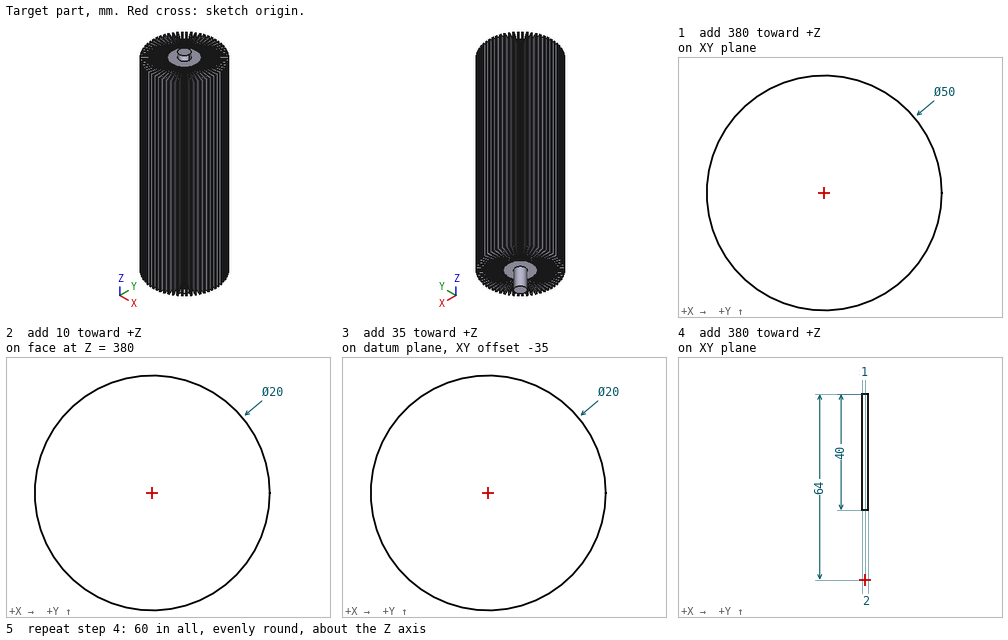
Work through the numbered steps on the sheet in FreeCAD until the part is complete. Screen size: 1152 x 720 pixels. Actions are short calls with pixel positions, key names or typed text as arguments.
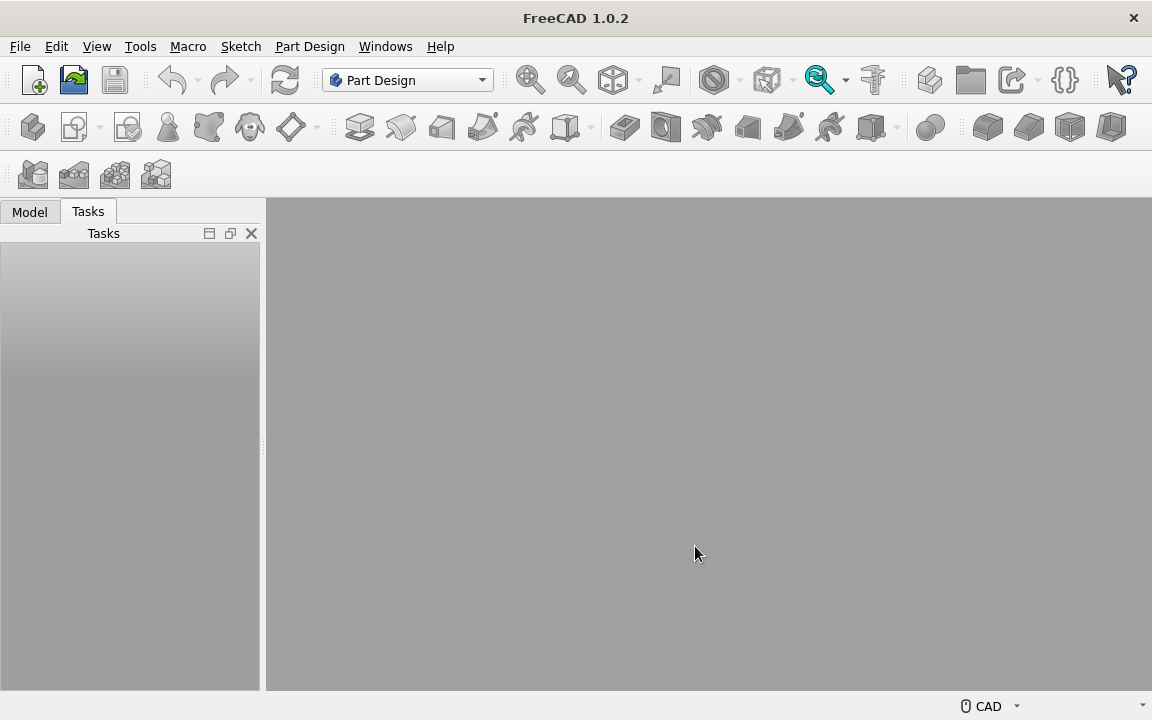
click(33, 80)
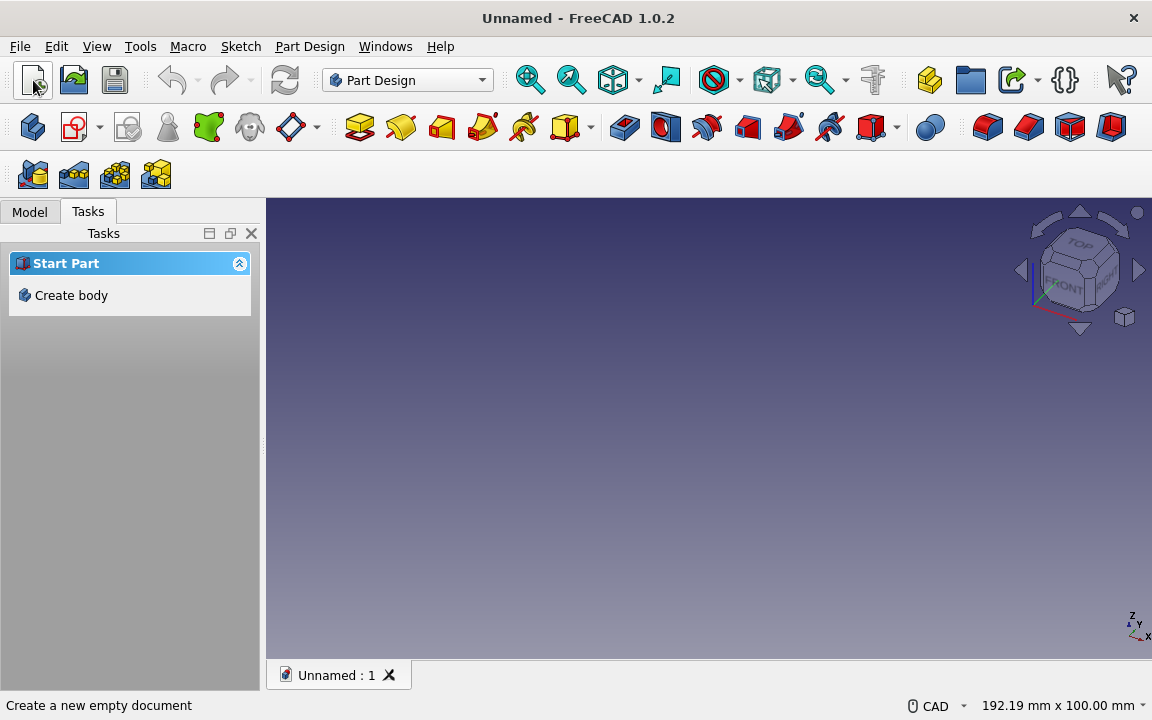
click(74, 128)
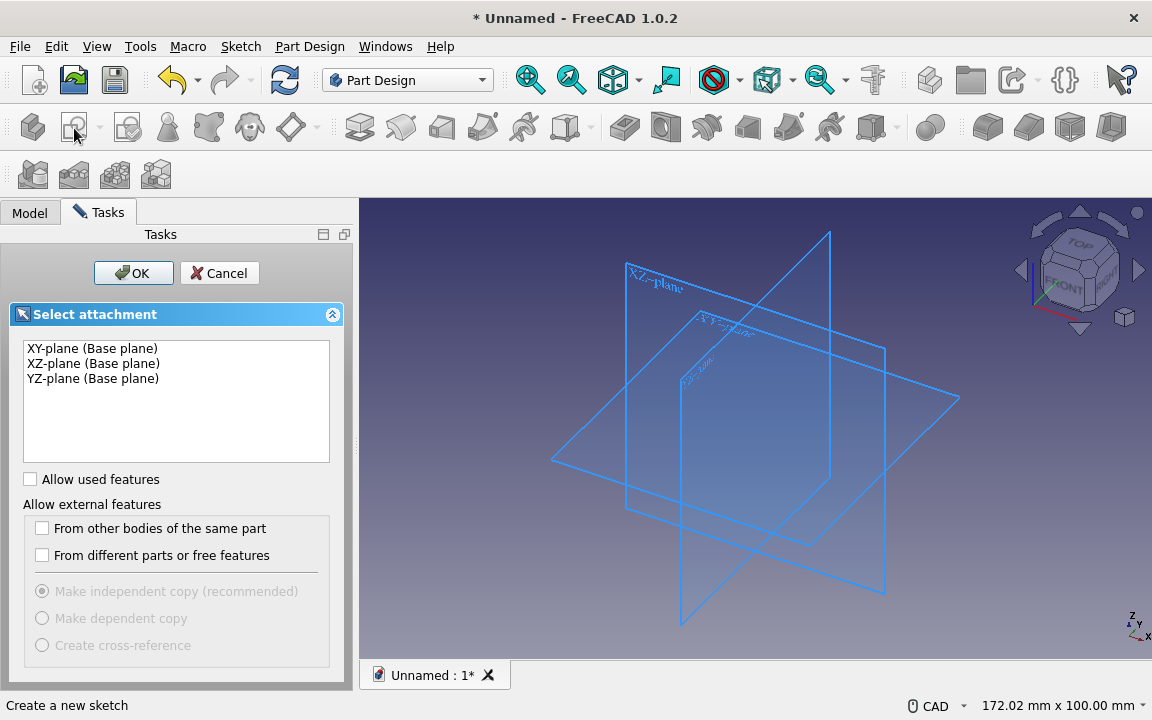
click(84, 348)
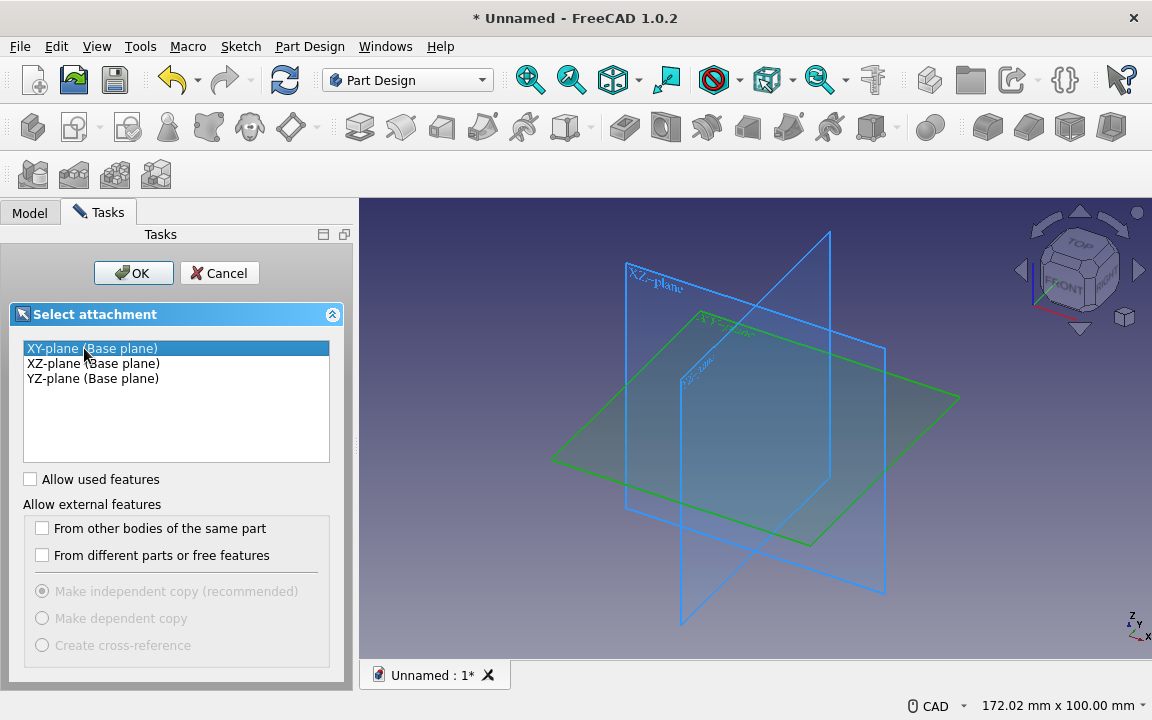
click(134, 273)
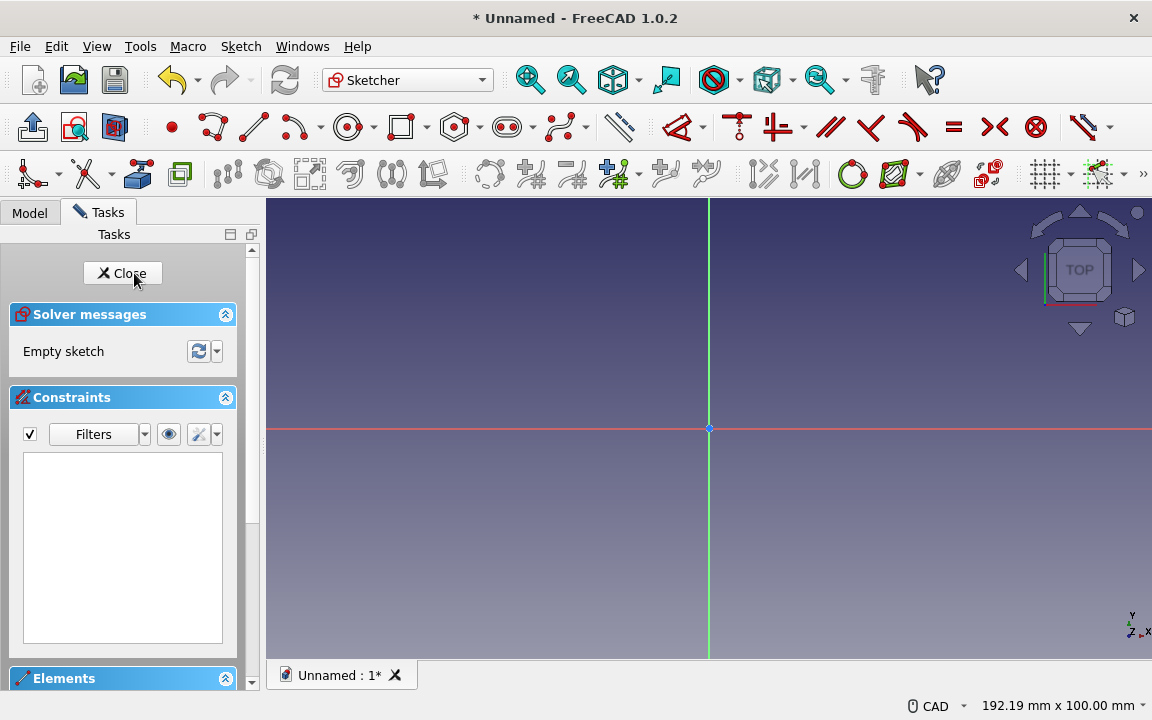
key(g)
key(c)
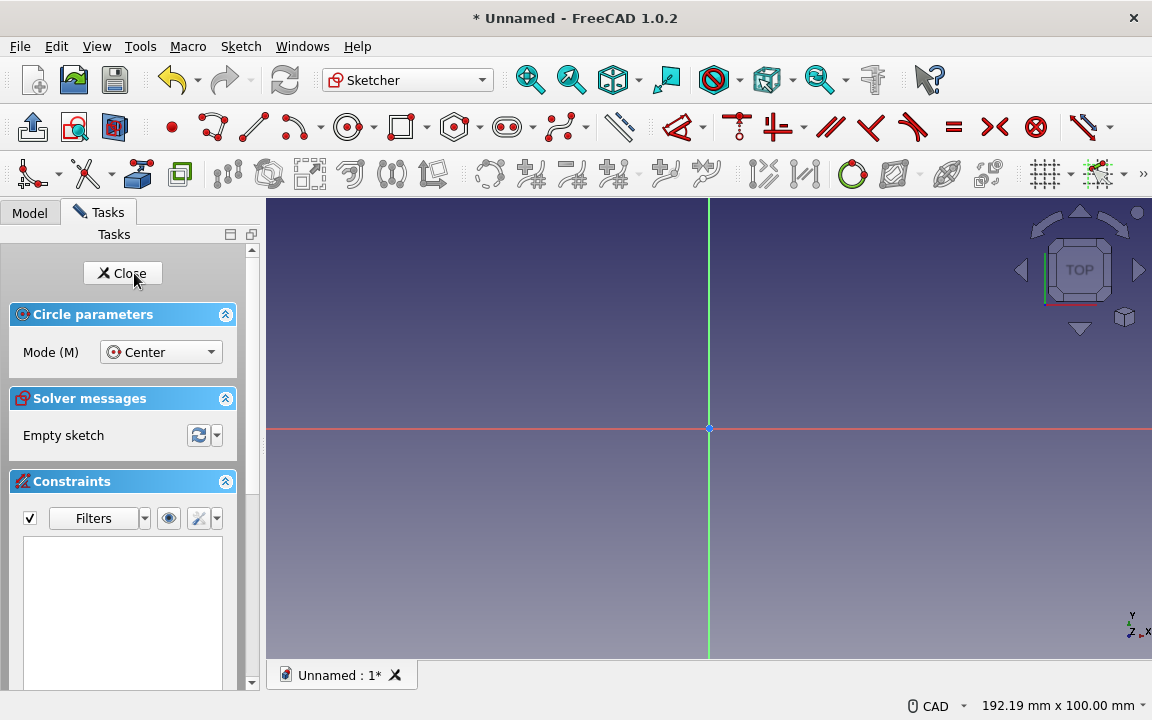
click(709, 428)
click(790, 347)
key(Escape)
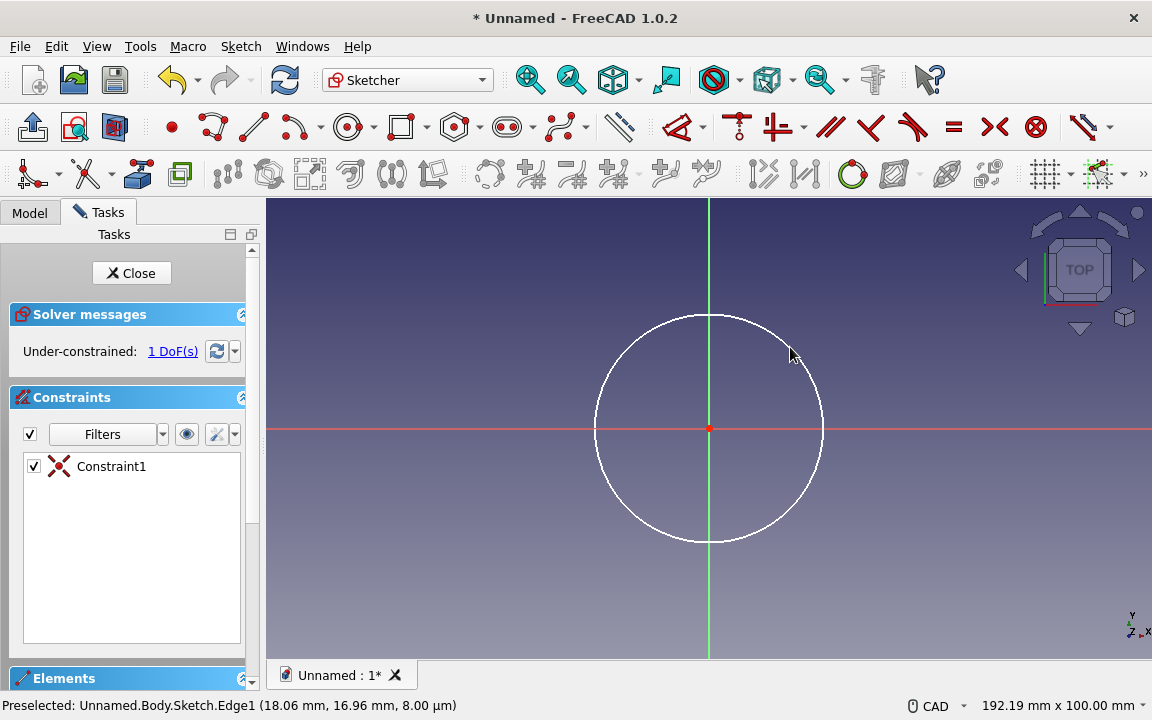
click(676, 128)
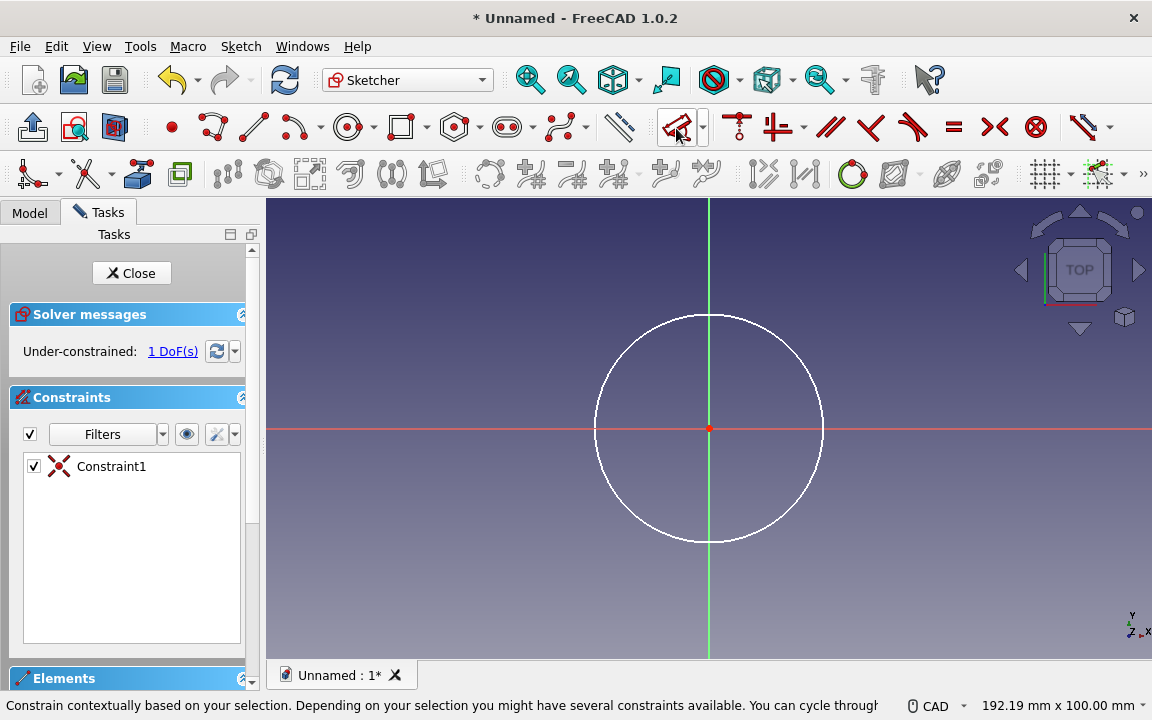
click(789, 347)
click(811, 324)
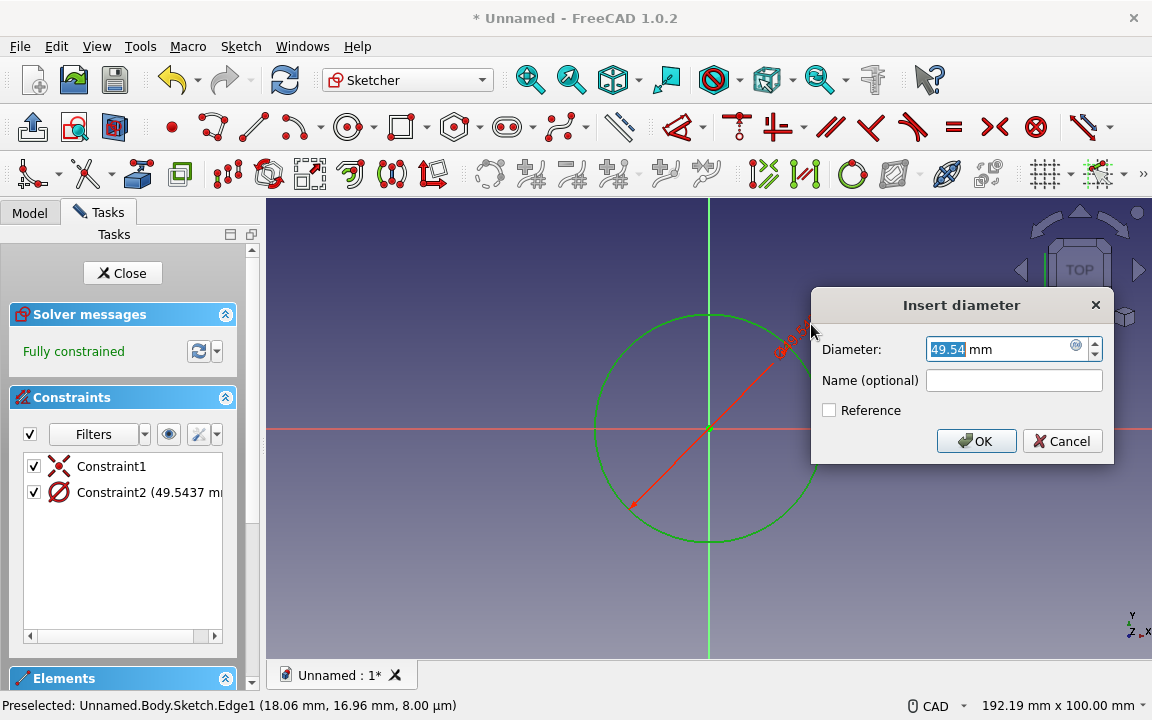
text(50)
key(Return)
key(Escape)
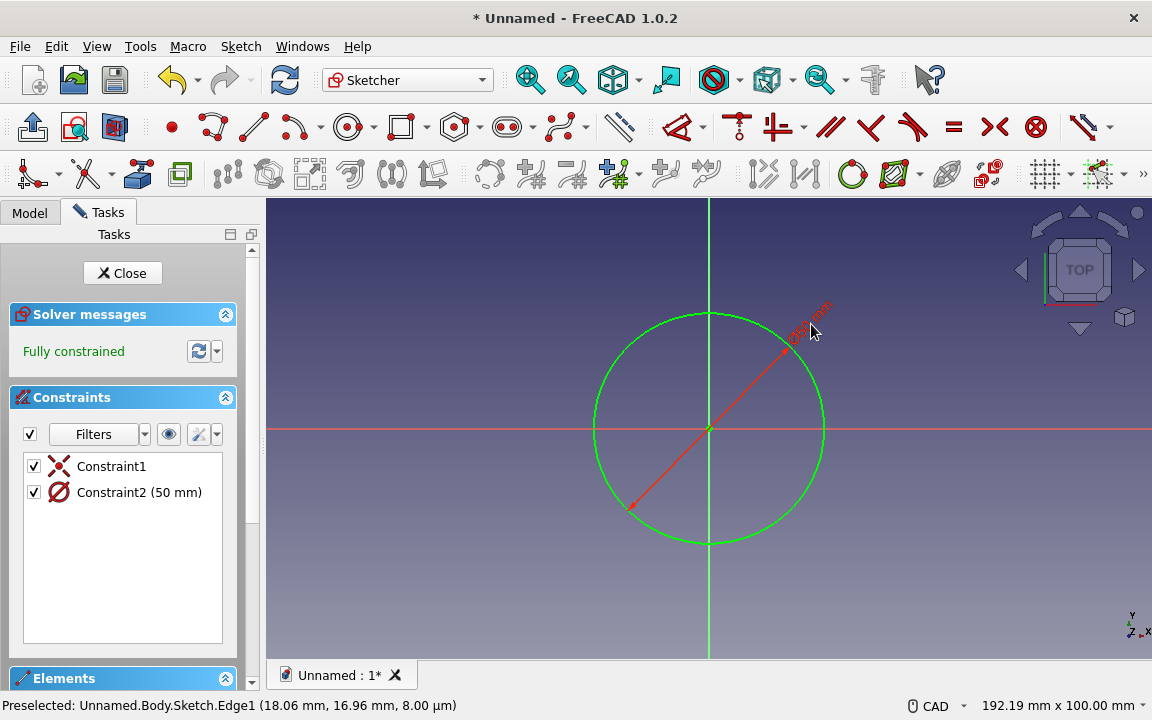
click(123, 273)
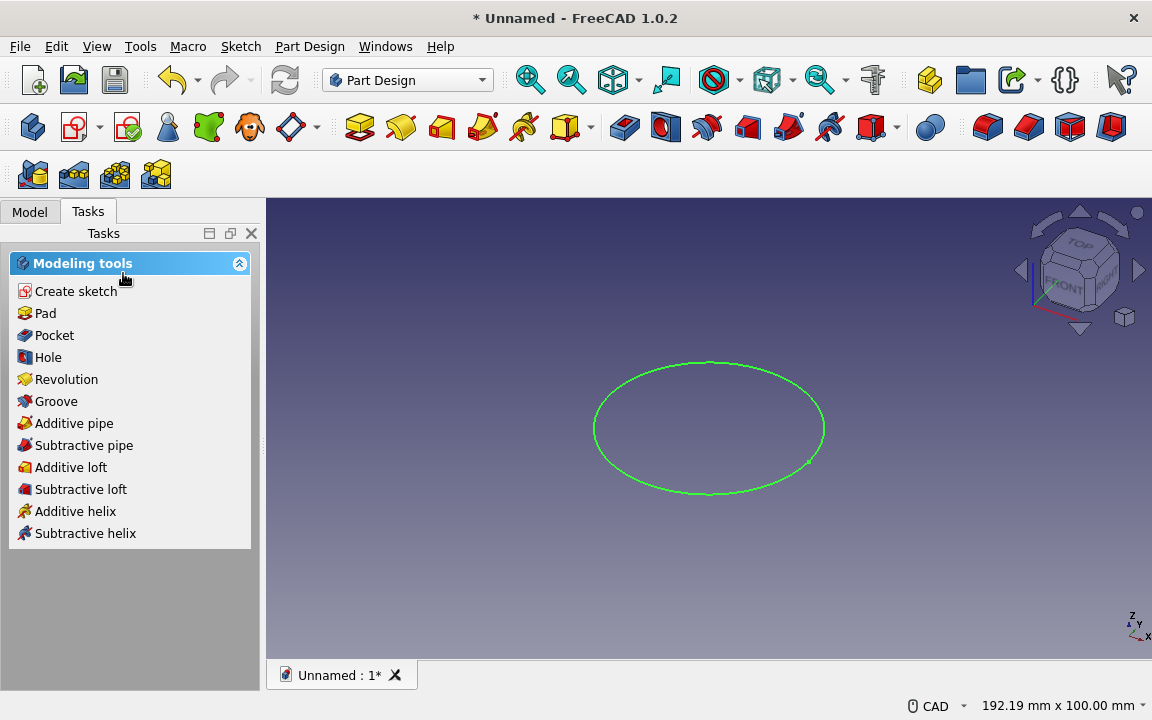
click(360, 128)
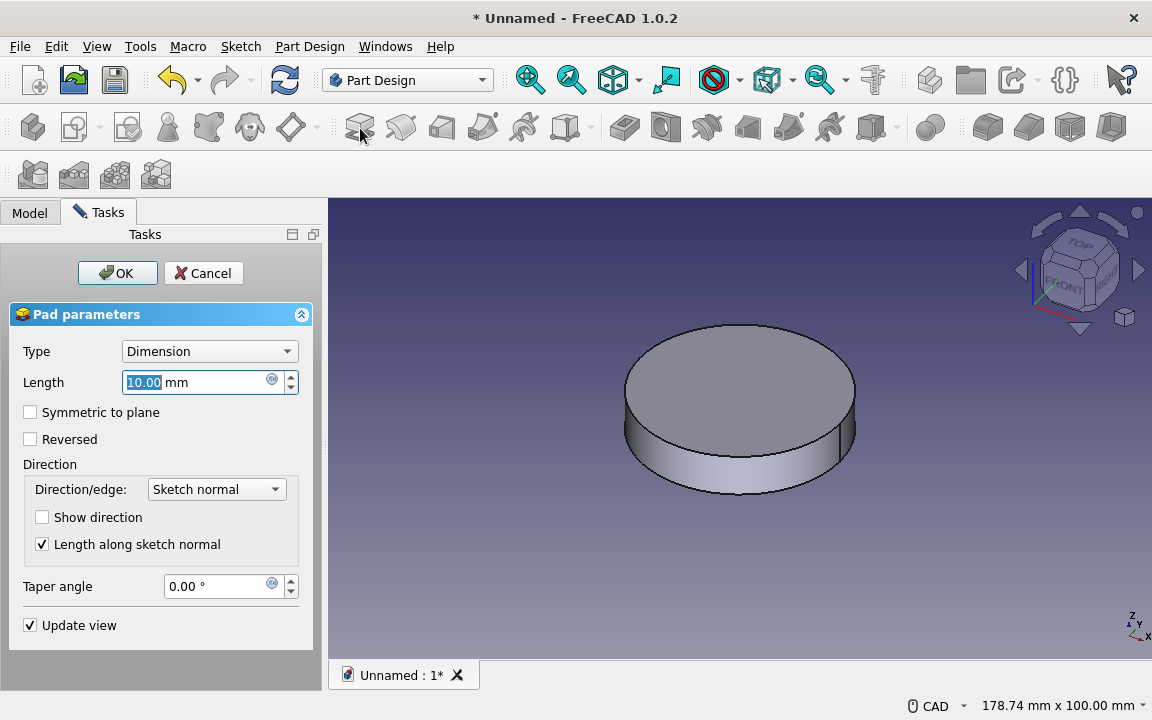
text(380)
key(Tab)